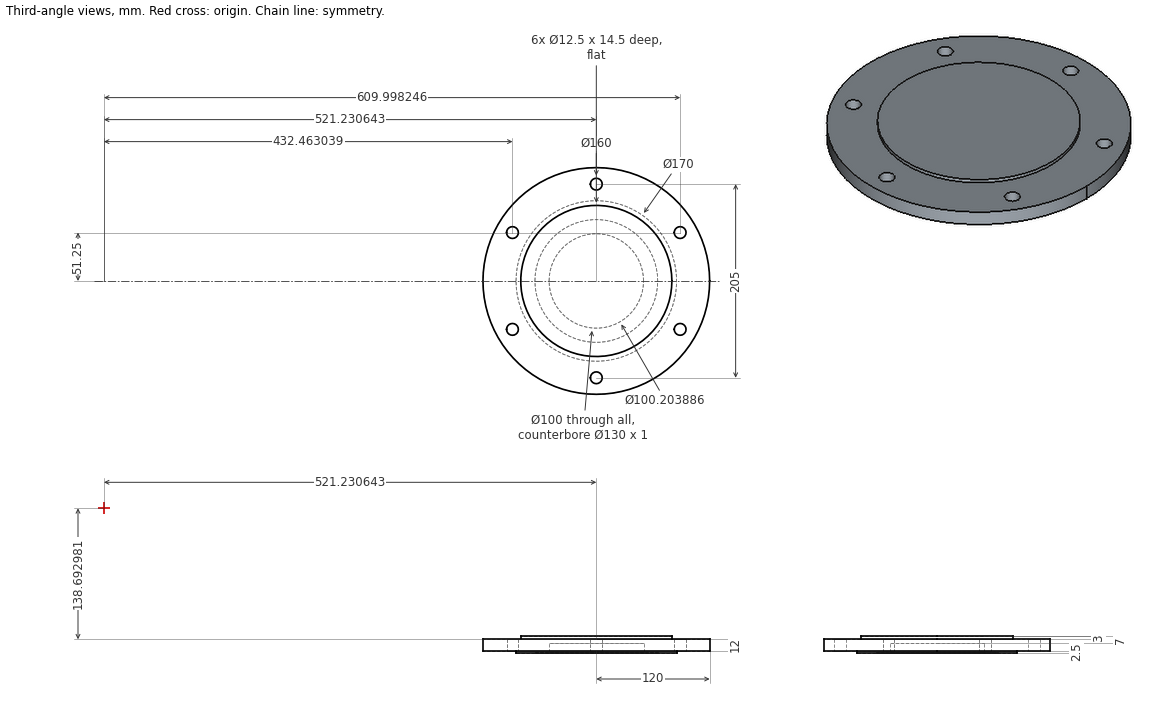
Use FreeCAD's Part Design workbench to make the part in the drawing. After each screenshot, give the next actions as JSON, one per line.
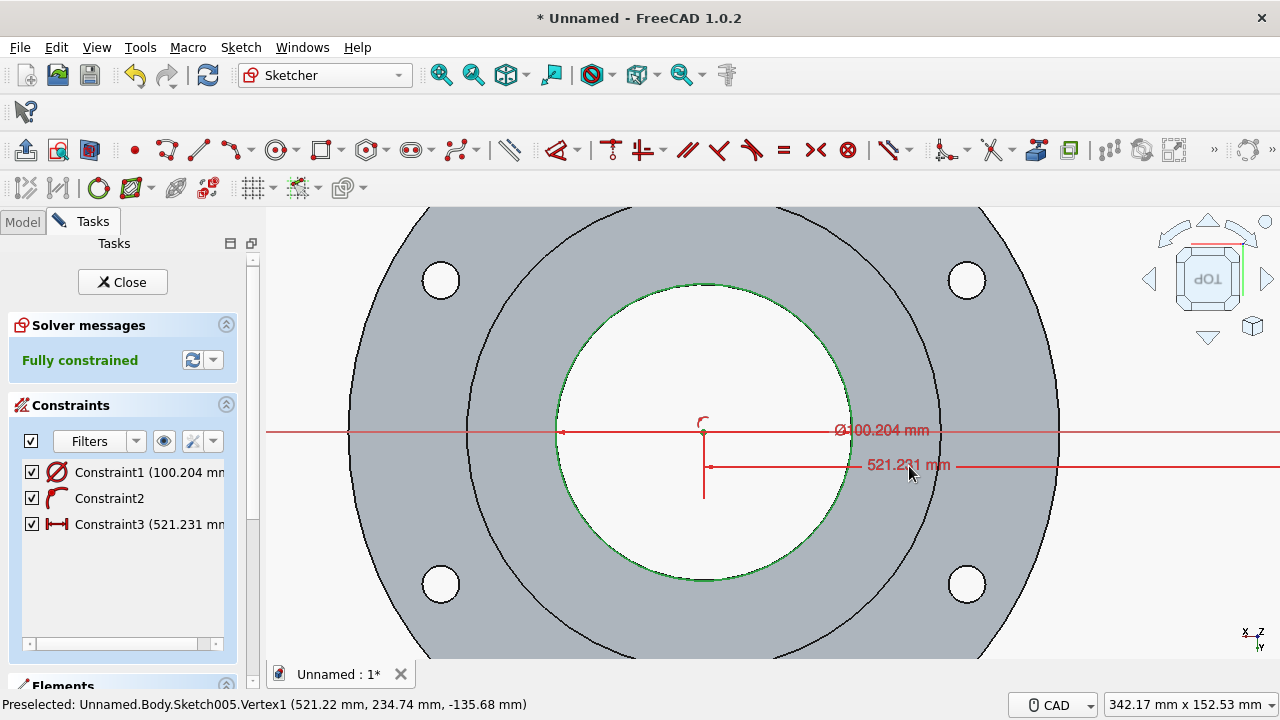
{"action": "left_click", "coordinate": [123, 282]}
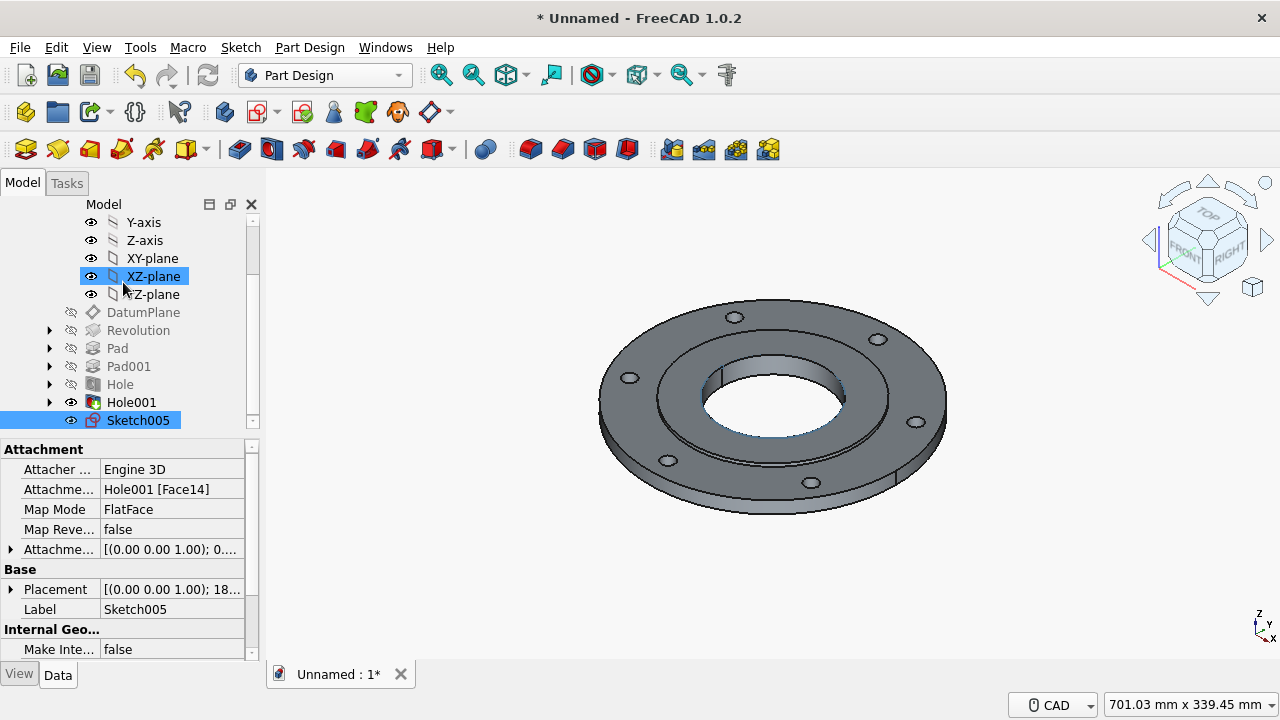
{"action": "left_click", "coordinate": [26, 150]}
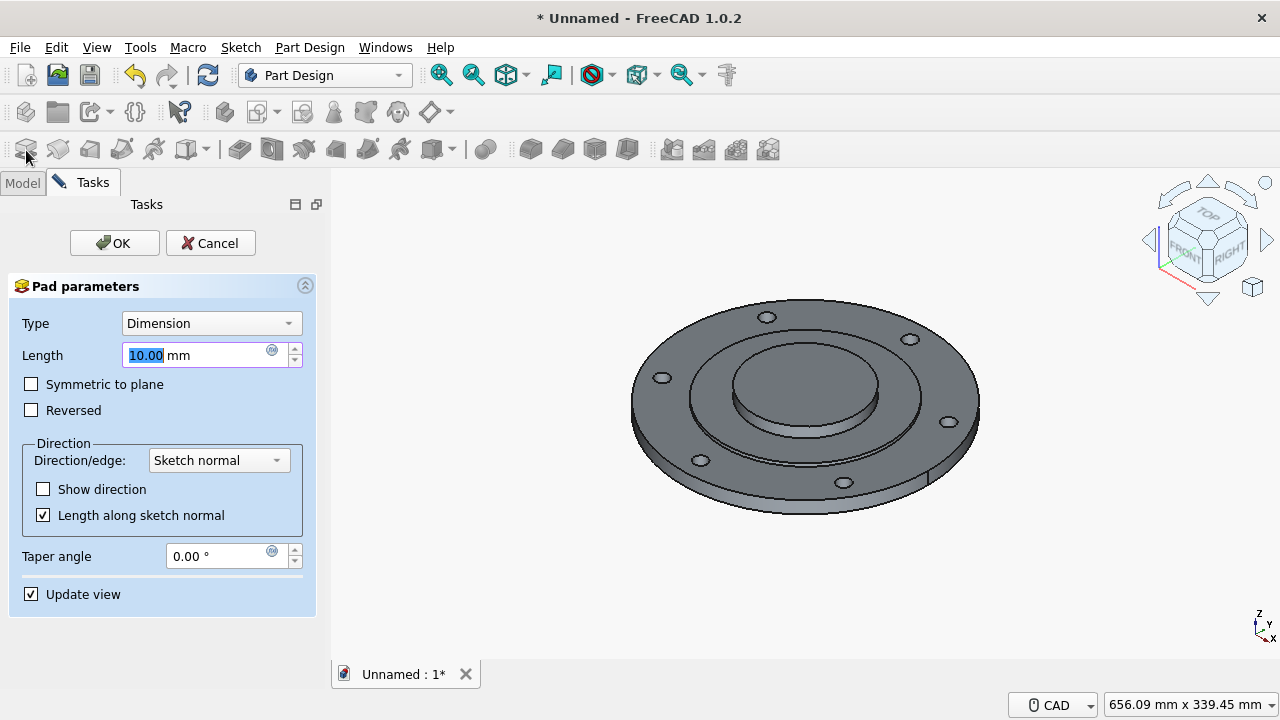
{"action": "type", "text": "7"}
{"action": "key", "text": "Tab"}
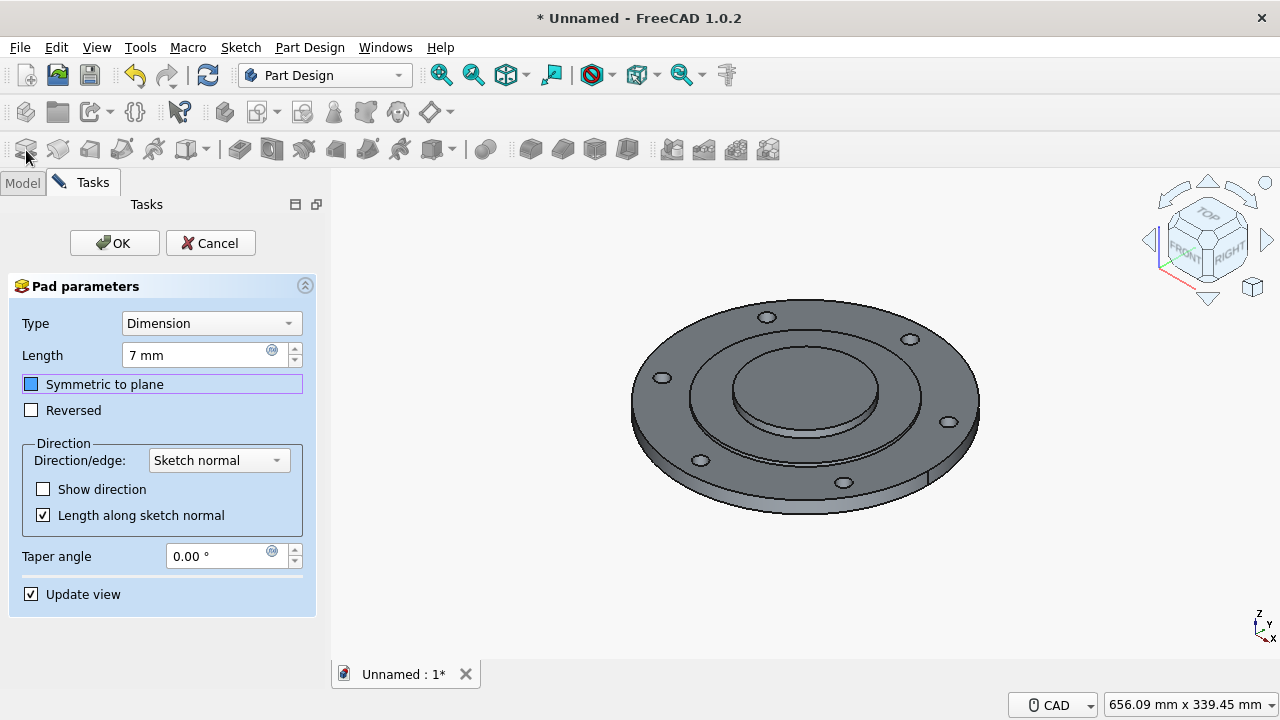
{"action": "left_click", "coordinate": [30, 410]}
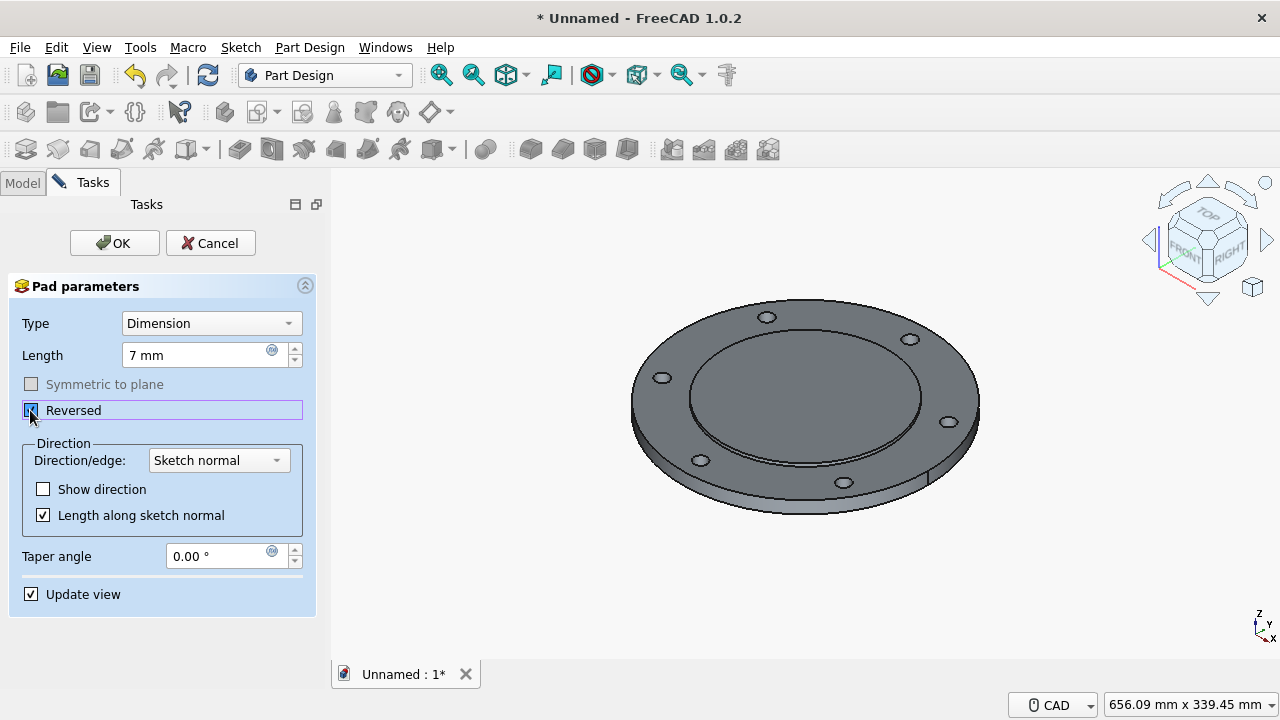
{"action": "left_click", "coordinate": [115, 243]}